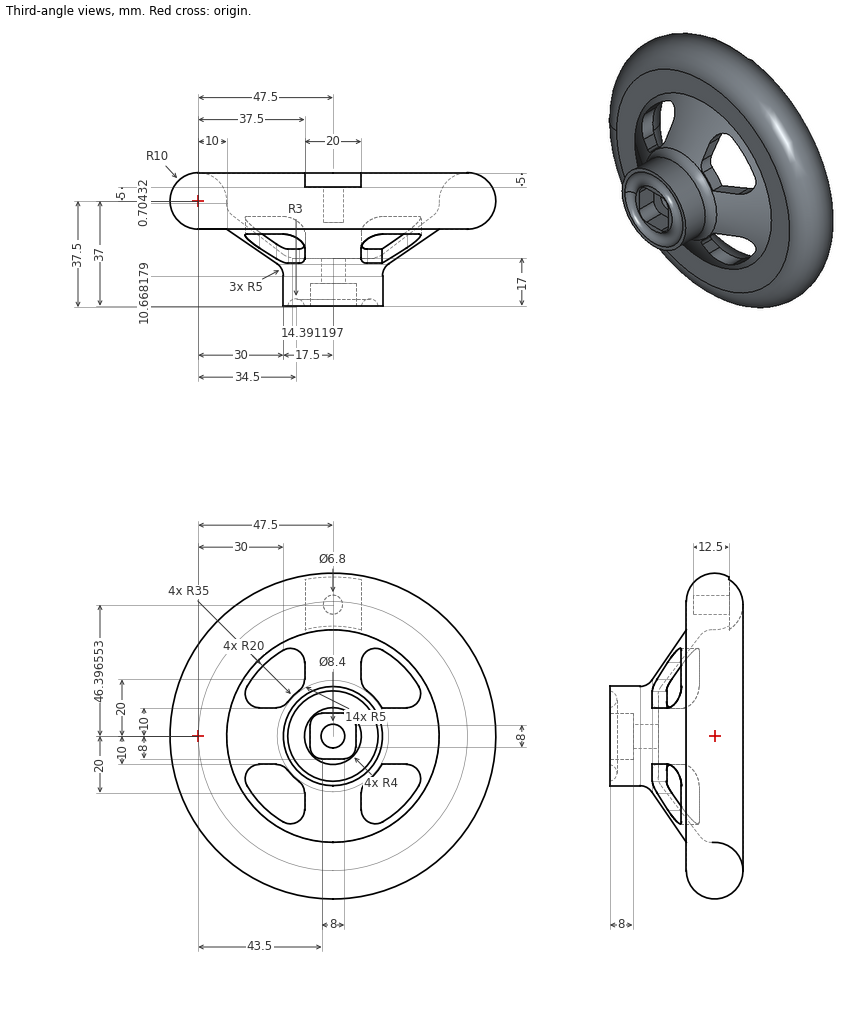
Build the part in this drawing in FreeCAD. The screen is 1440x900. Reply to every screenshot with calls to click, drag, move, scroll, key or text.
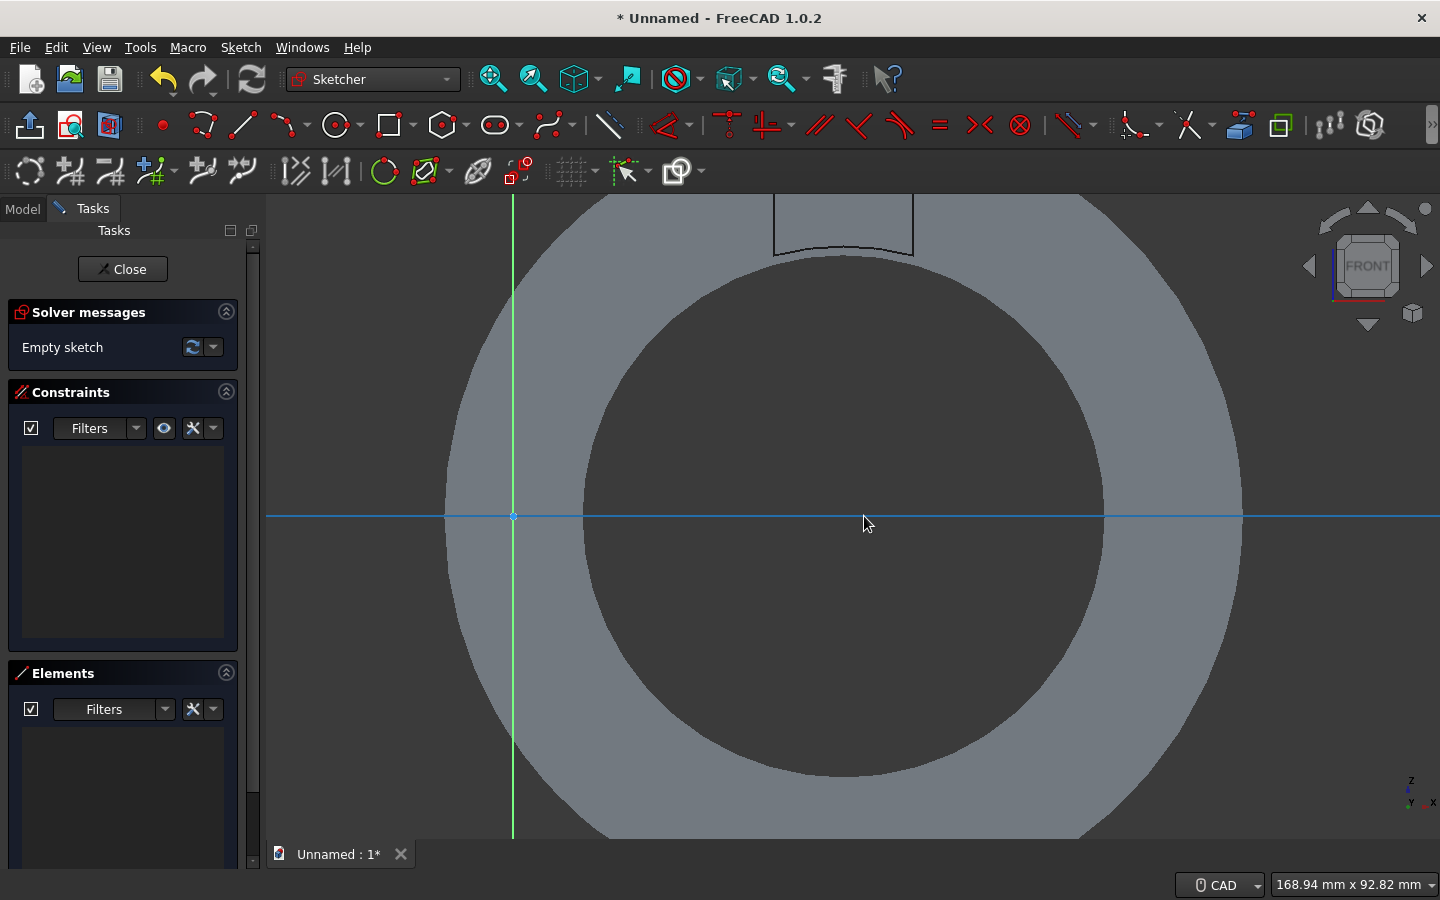
click(244, 126)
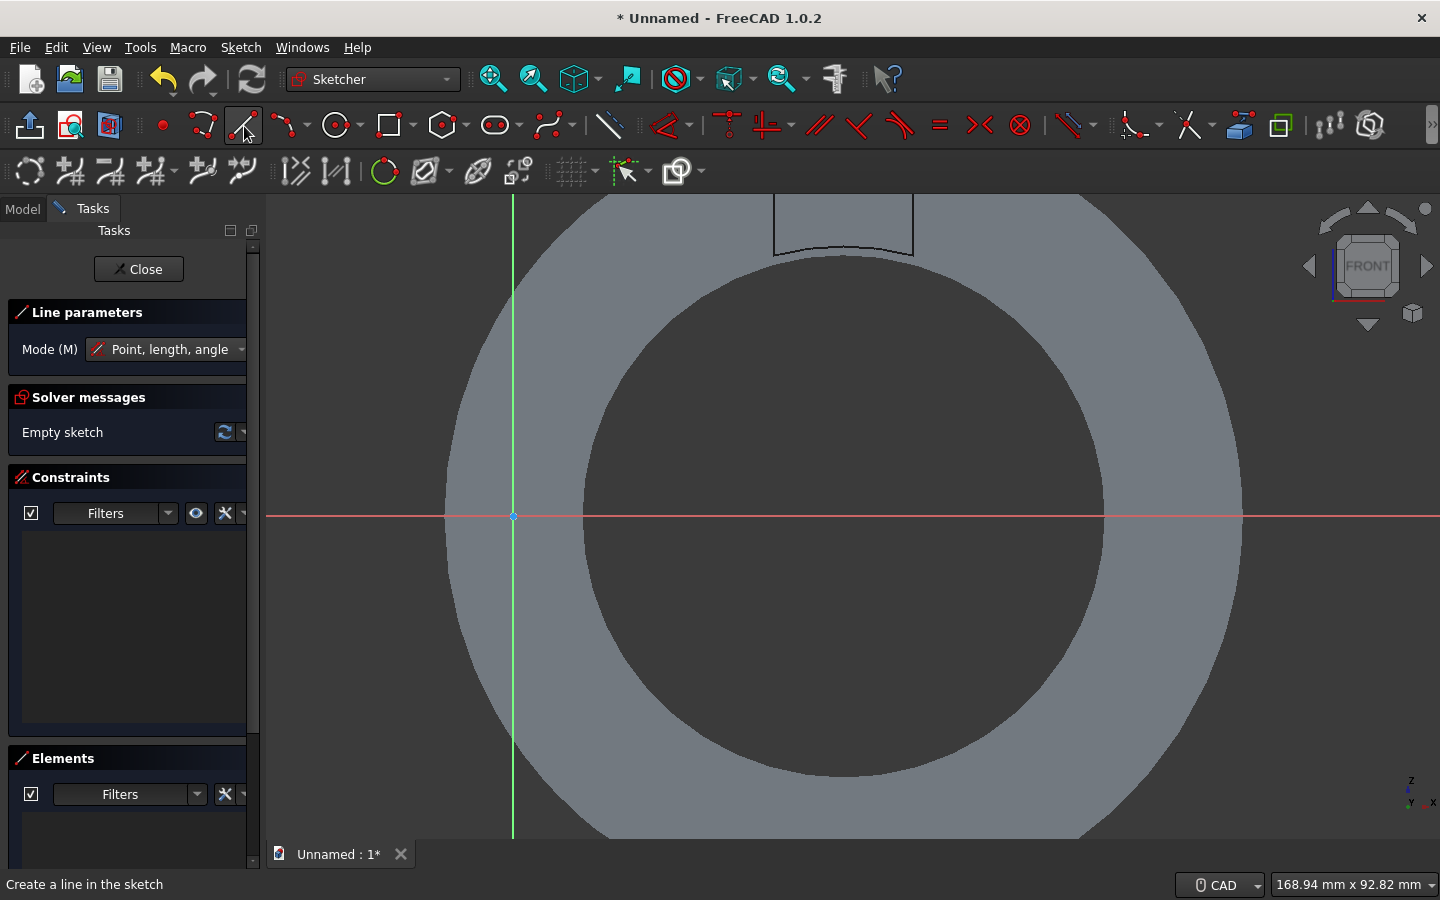
click(705, 447)
click(663, 447)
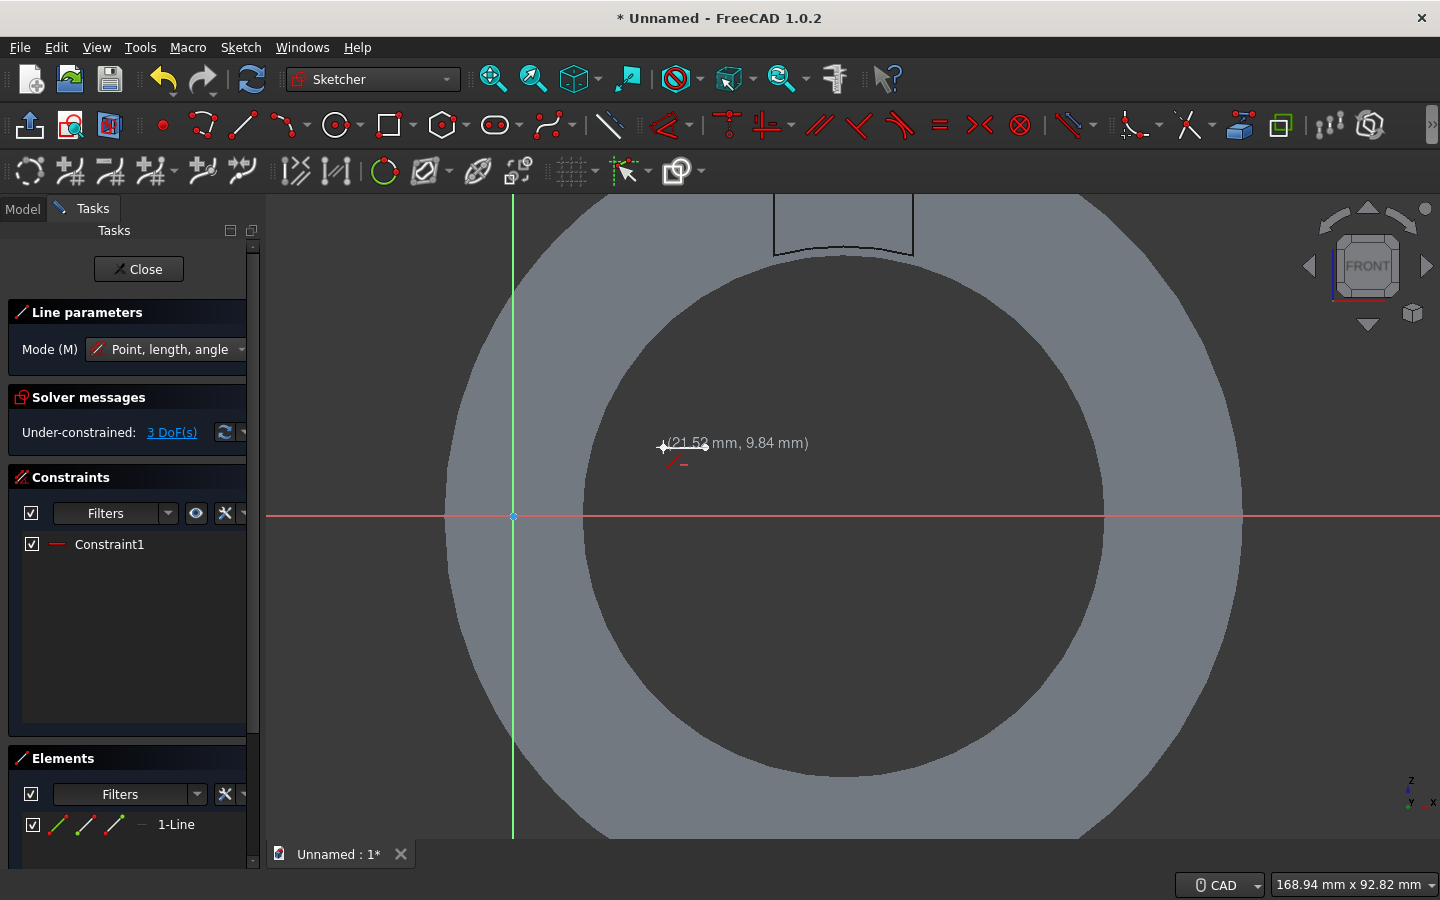
click(774, 336)
click(774, 377)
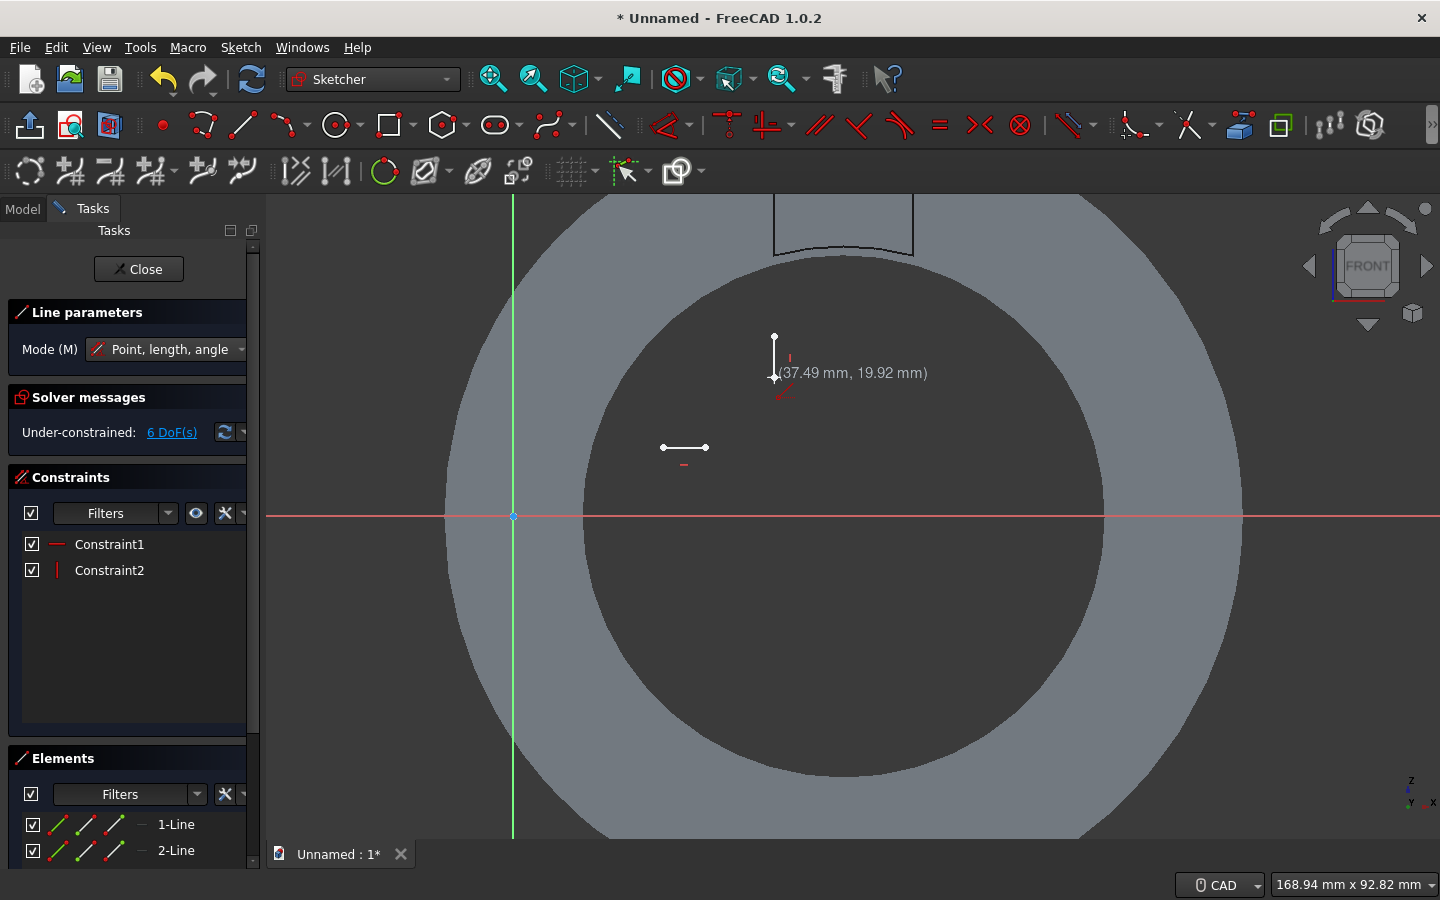
click(284, 126)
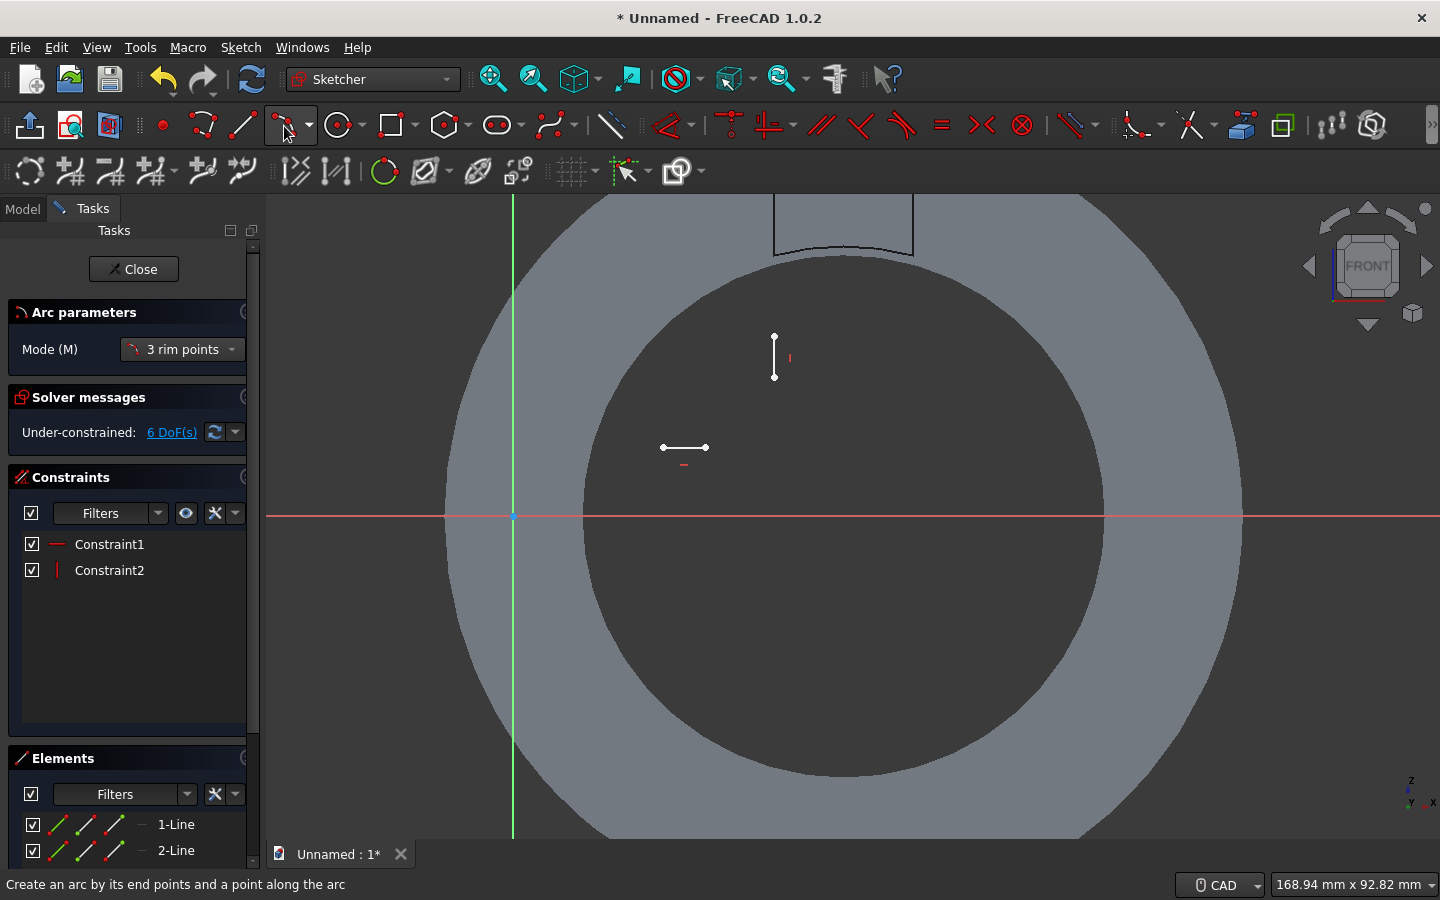
click(663, 448)
click(633, 395)
click(633, 430)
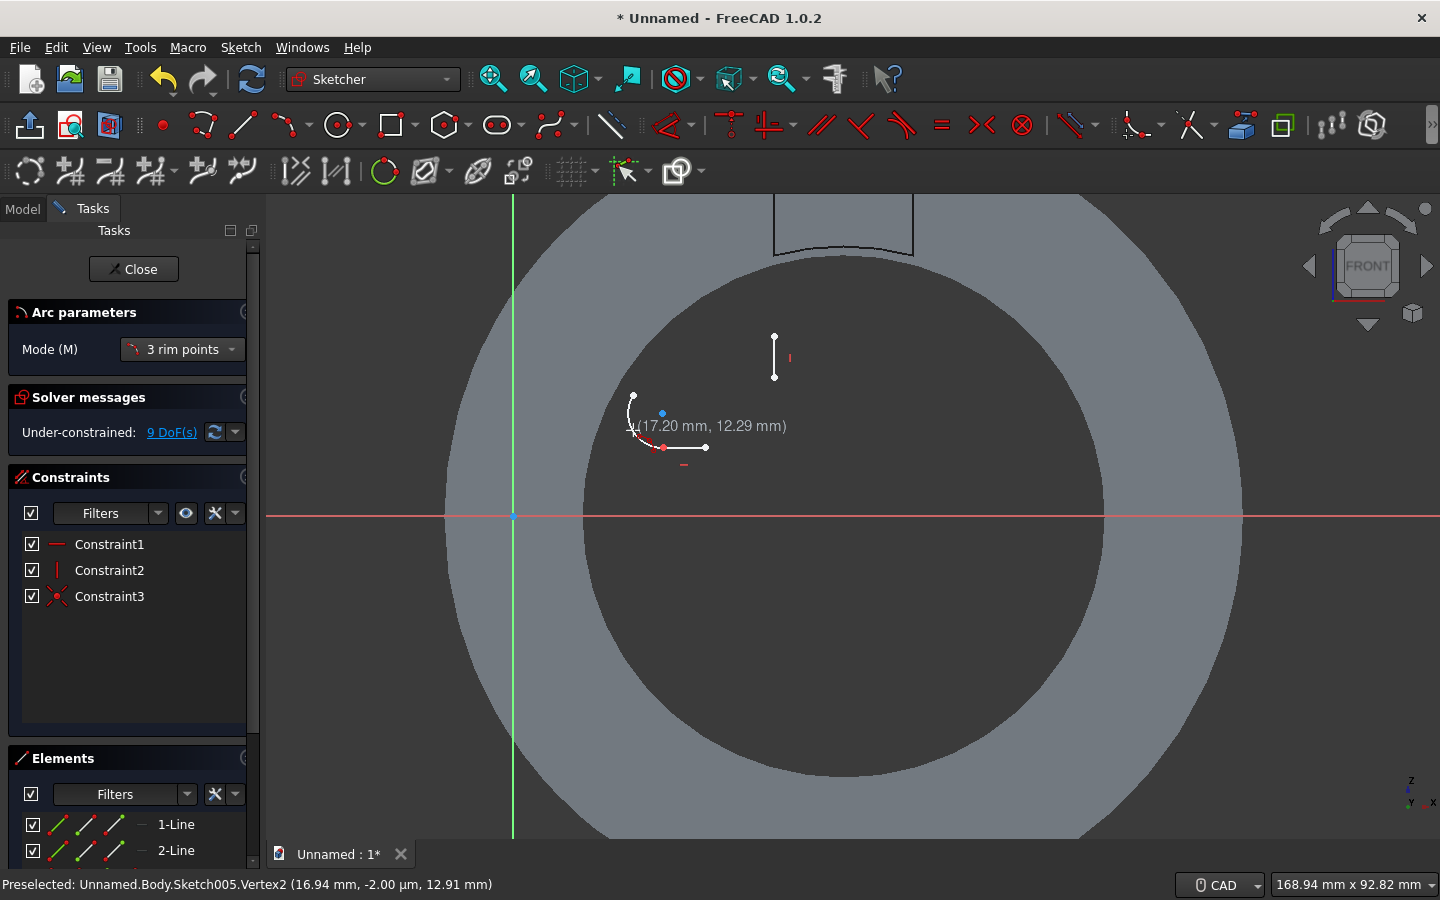
click(633, 396)
click(722, 306)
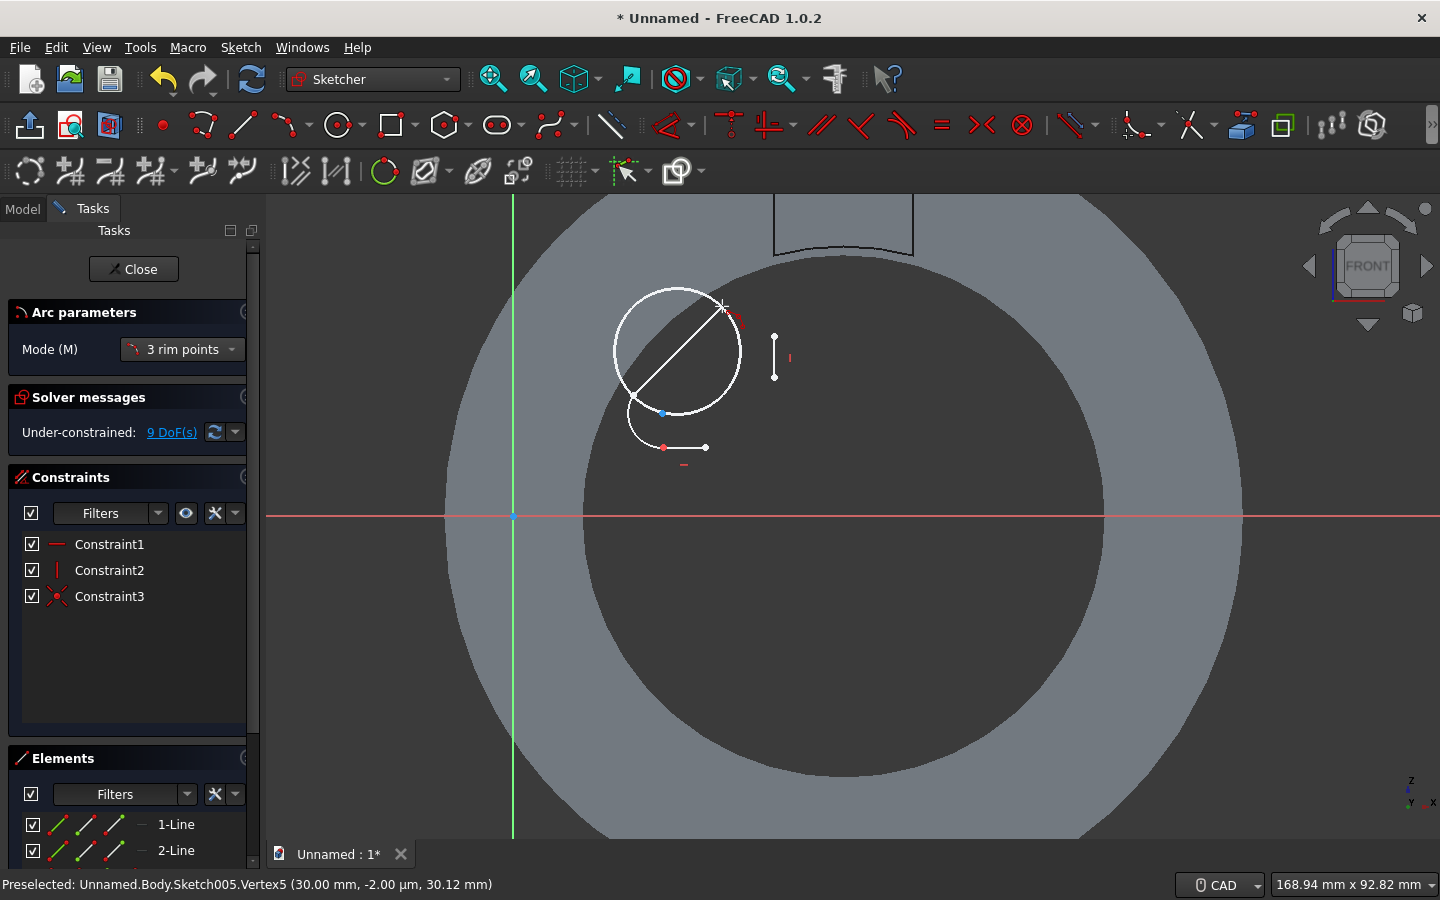
scroll(672, 344, up, 4)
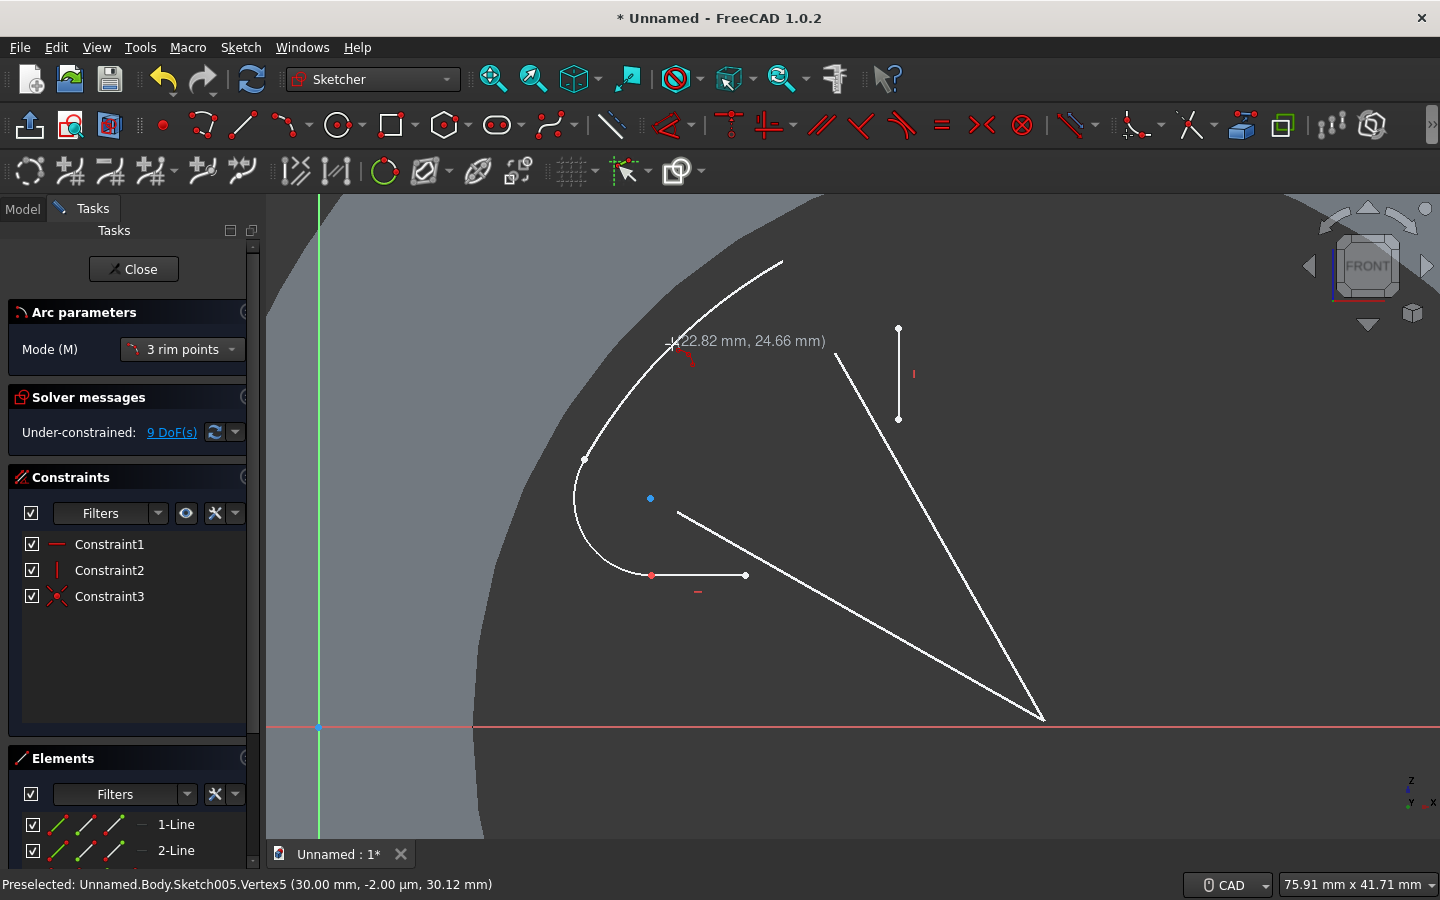
click(671, 345)